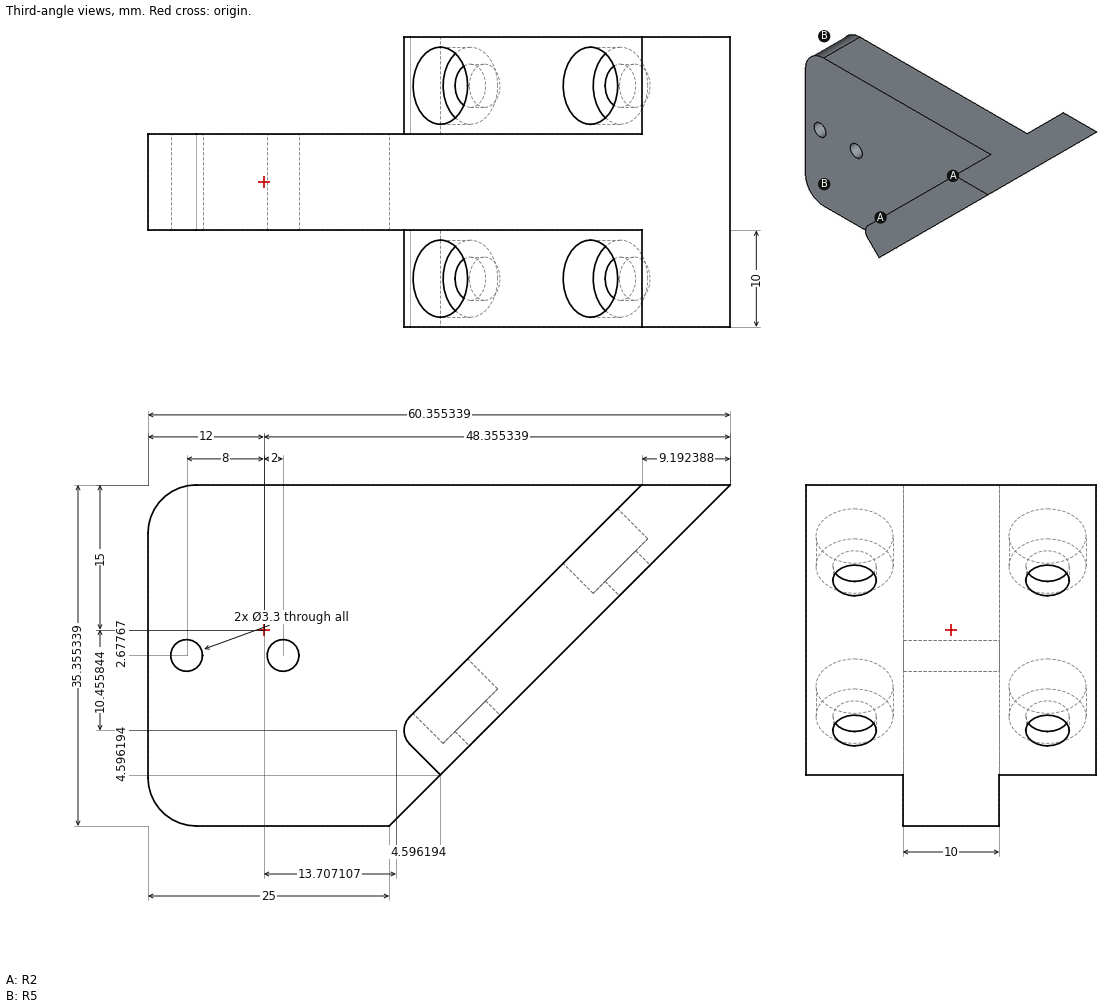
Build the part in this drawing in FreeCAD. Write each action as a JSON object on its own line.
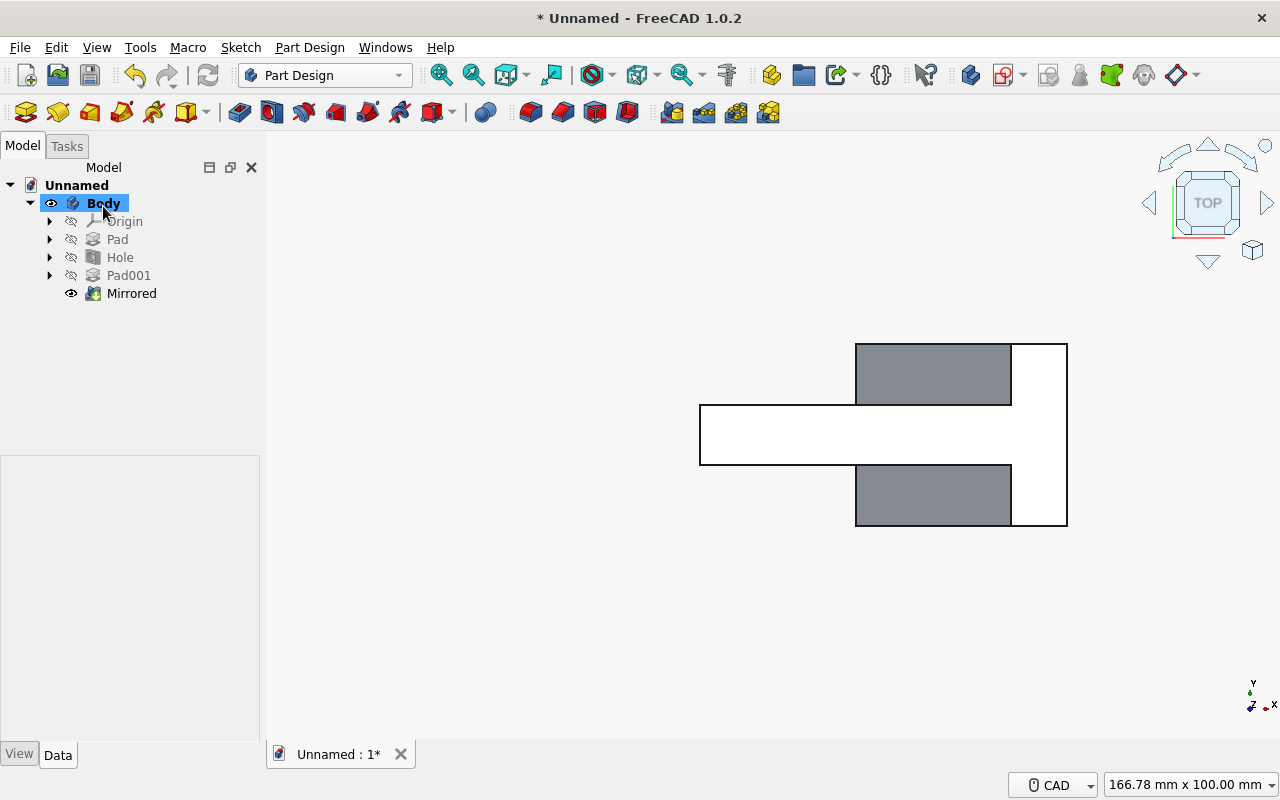
{"action": "left_click", "coordinate": [442, 76]}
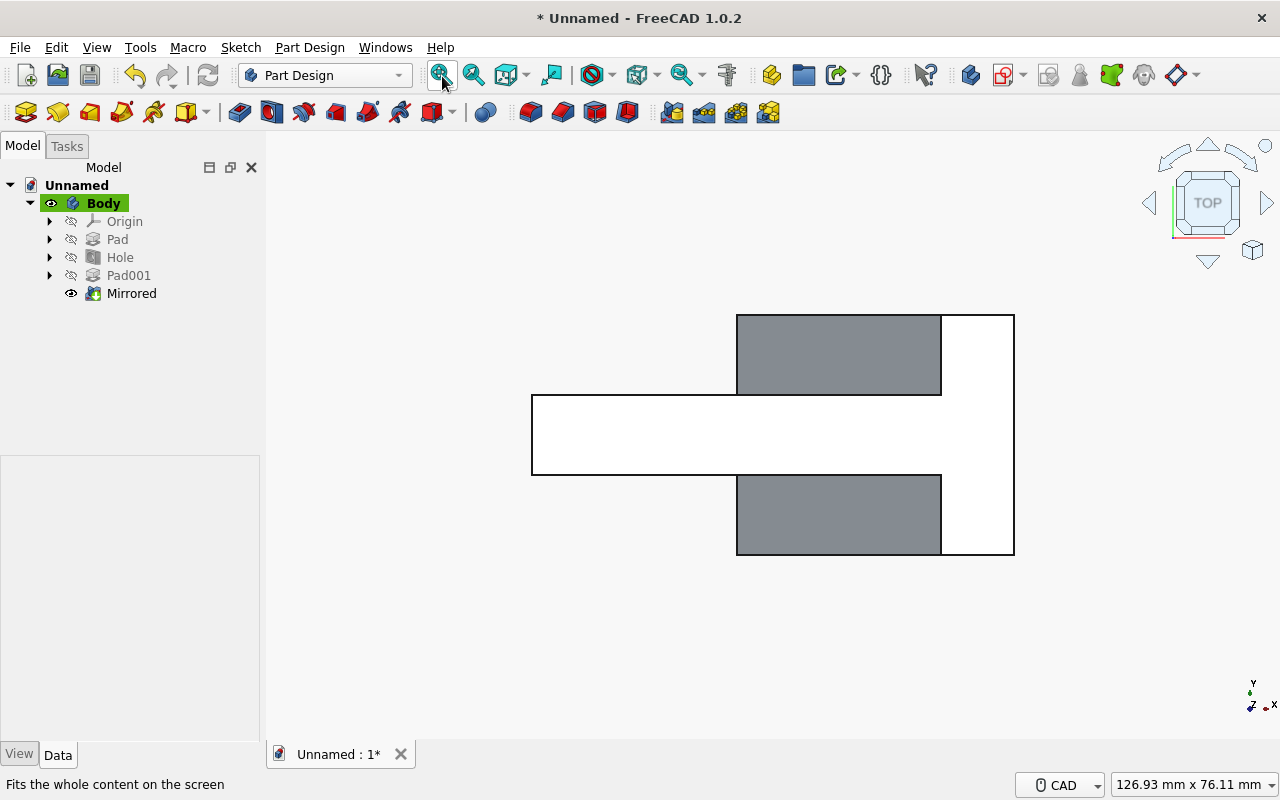
{"action": "left_click", "coordinate": [897, 354]}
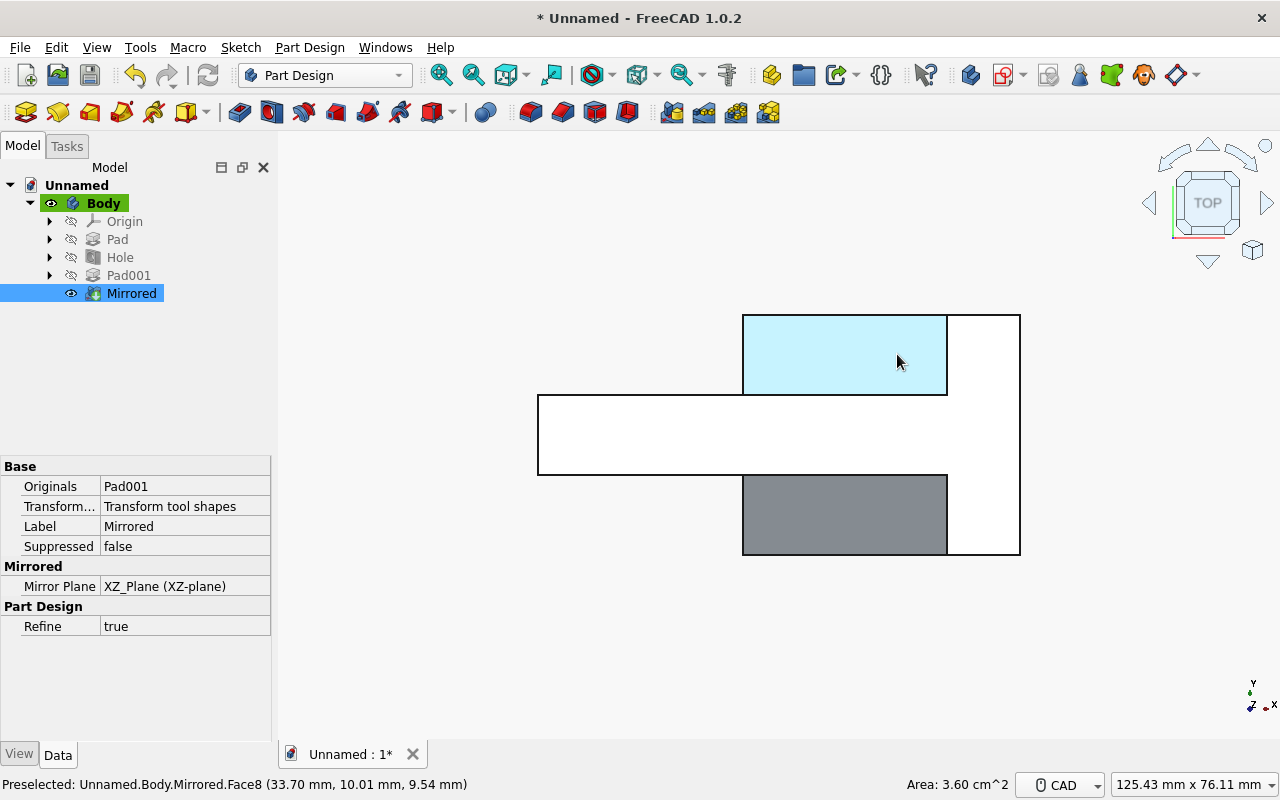
{"action": "left_click", "coordinate": [1004, 76]}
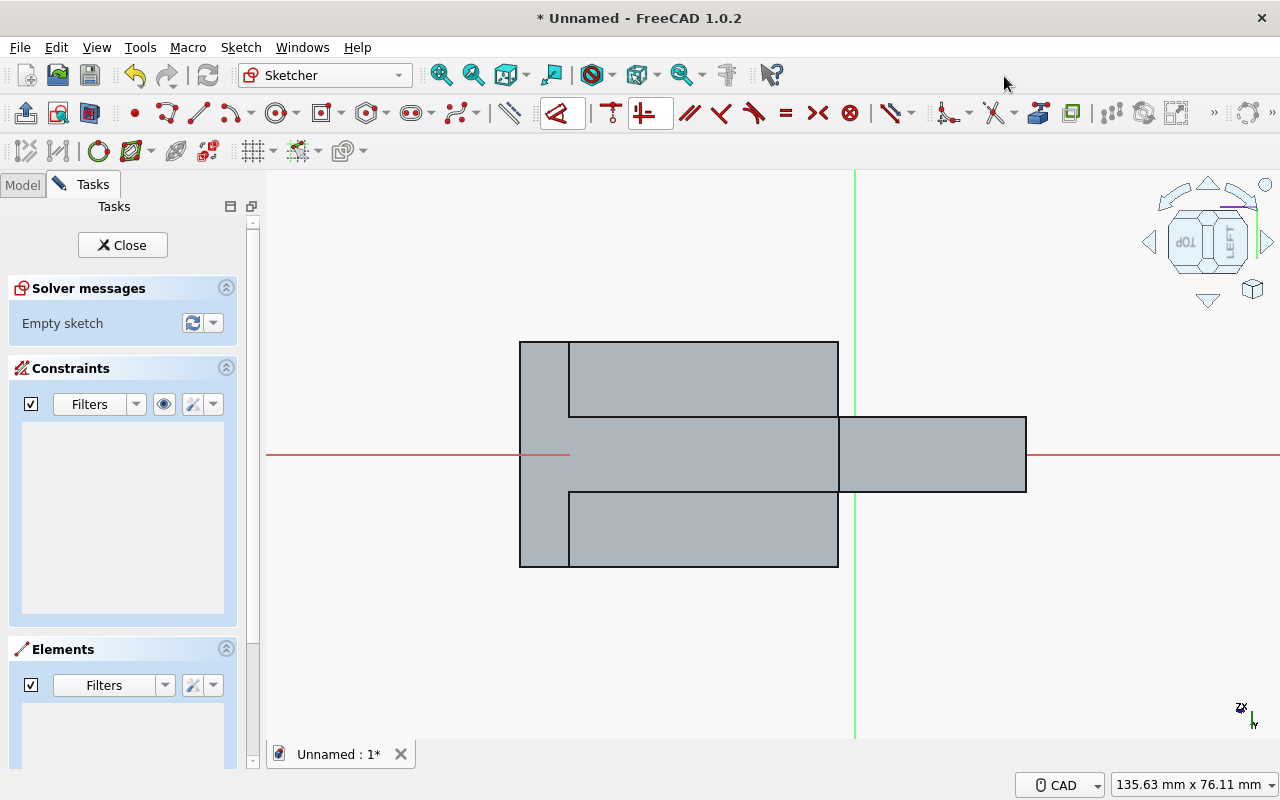
{"action": "left_click", "coordinate": [90, 114]}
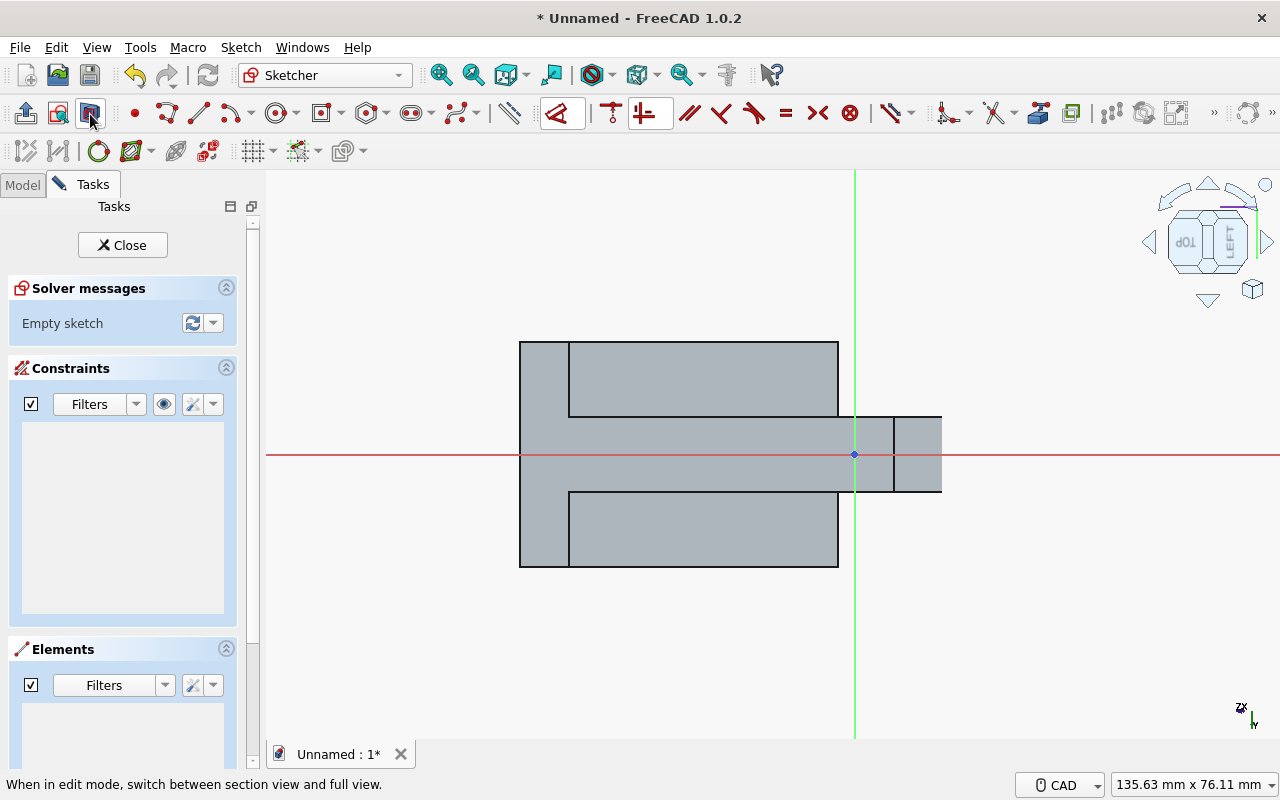
{"action": "scroll", "coordinate": [764, 454], "scroll_direction": "up", "scroll_amount": 3}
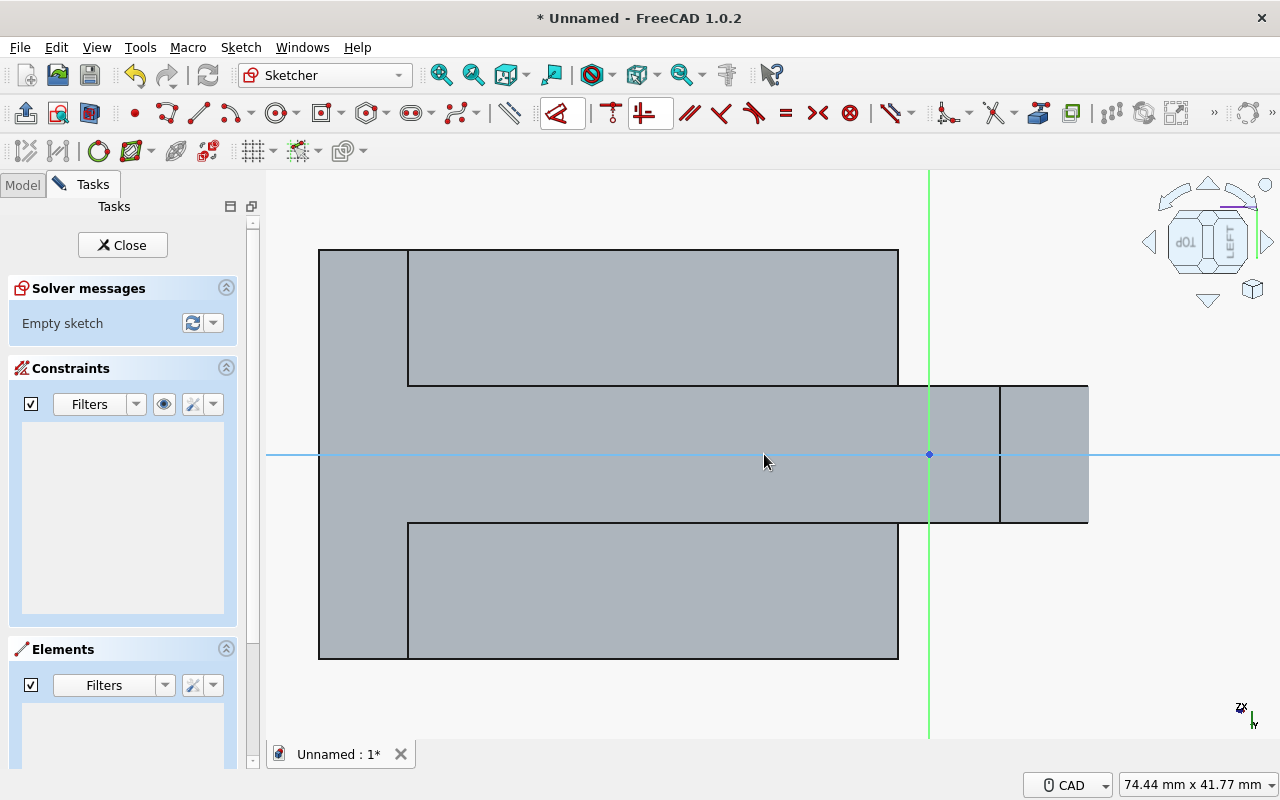
{"action": "left_click", "coordinate": [276, 114]}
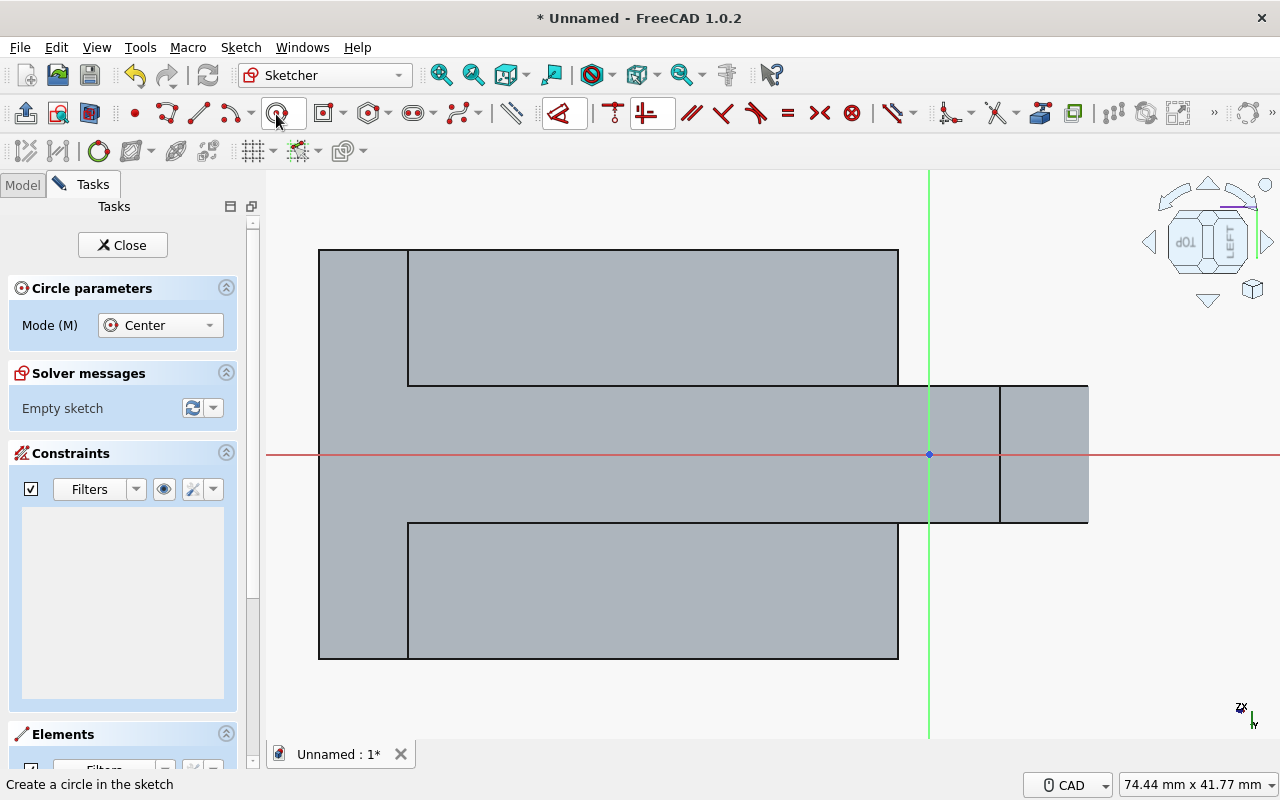
{"action": "left_click", "coordinate": [809, 591]}
{"action": "left_click", "coordinate": [831, 569]}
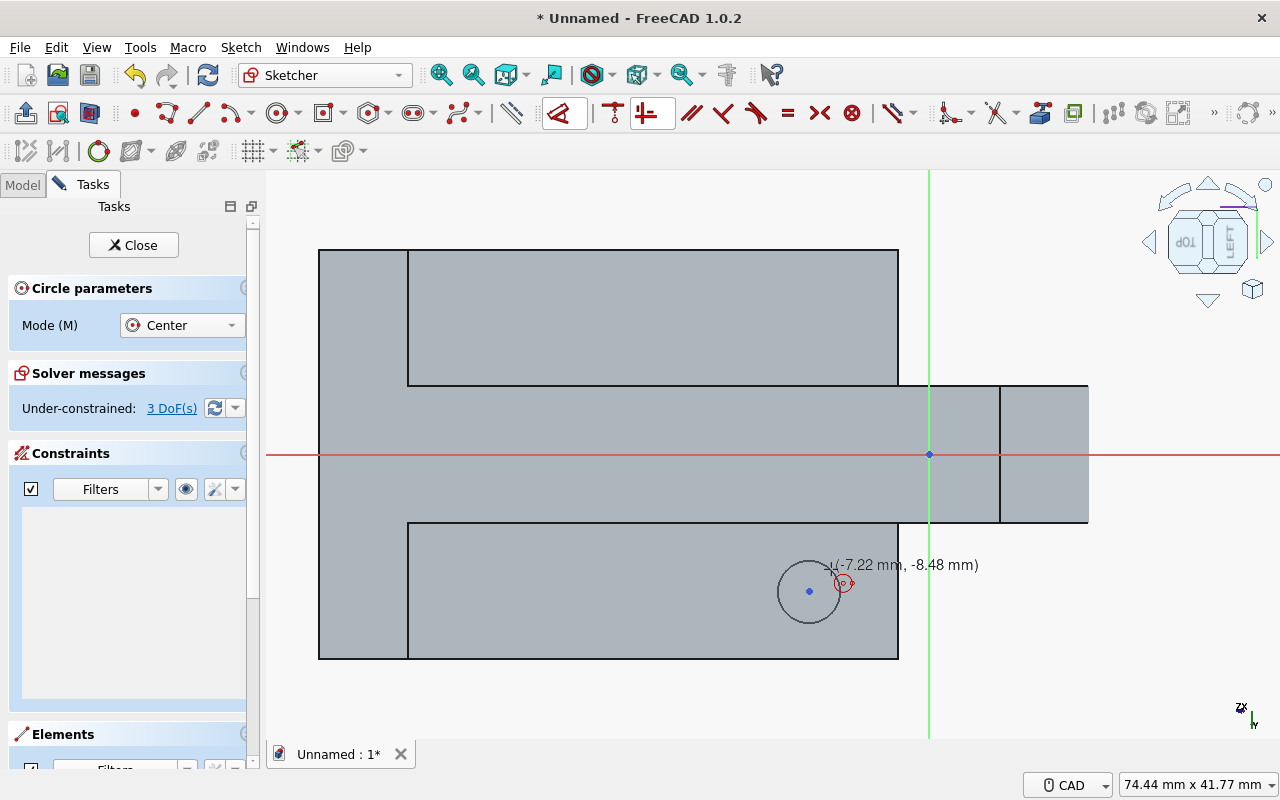
{"action": "left_click", "coordinate": [510, 591]}
{"action": "left_click", "coordinate": [531, 569]}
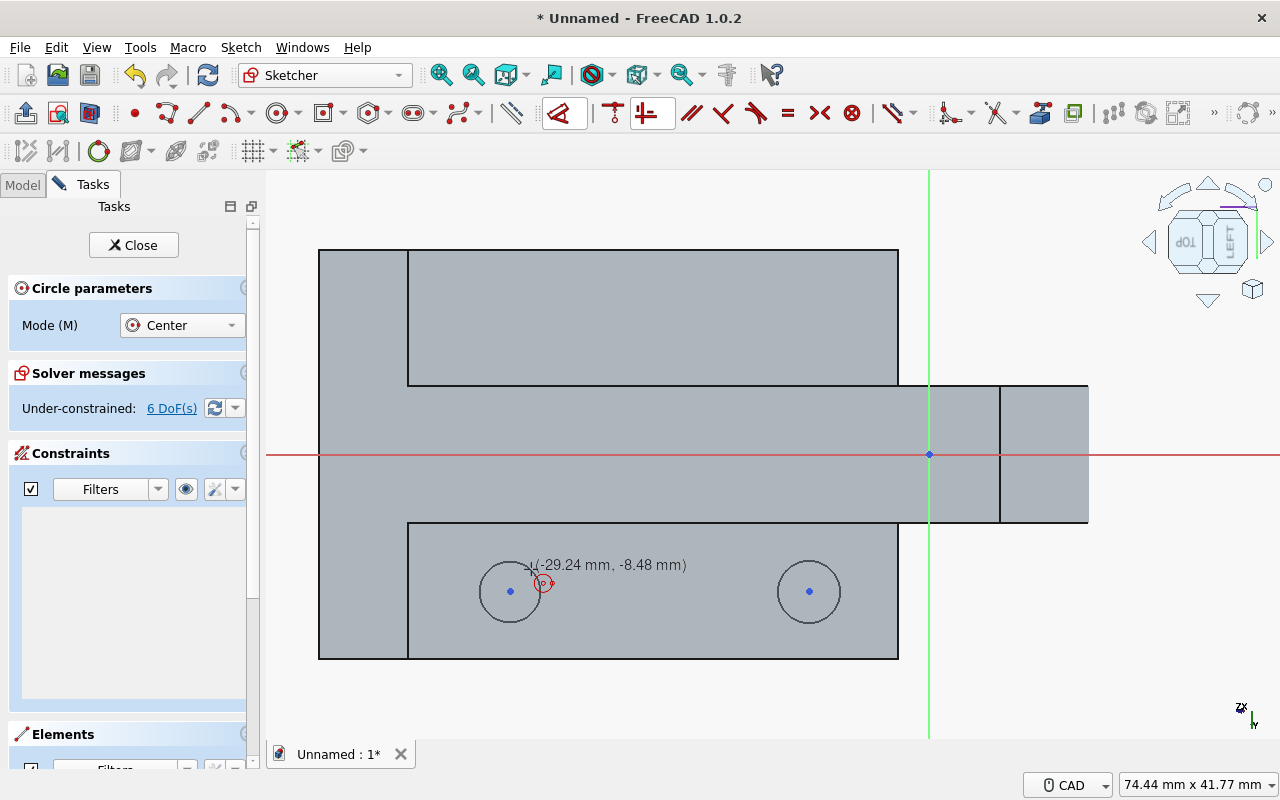
{"action": "left_click", "coordinate": [809, 318]}
{"action": "left_click", "coordinate": [831, 297]}